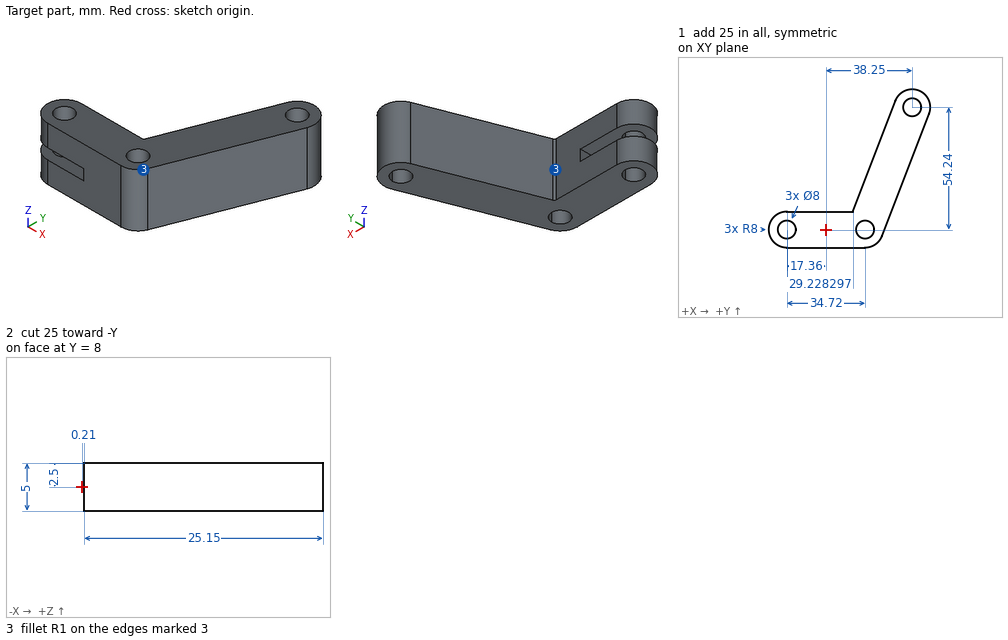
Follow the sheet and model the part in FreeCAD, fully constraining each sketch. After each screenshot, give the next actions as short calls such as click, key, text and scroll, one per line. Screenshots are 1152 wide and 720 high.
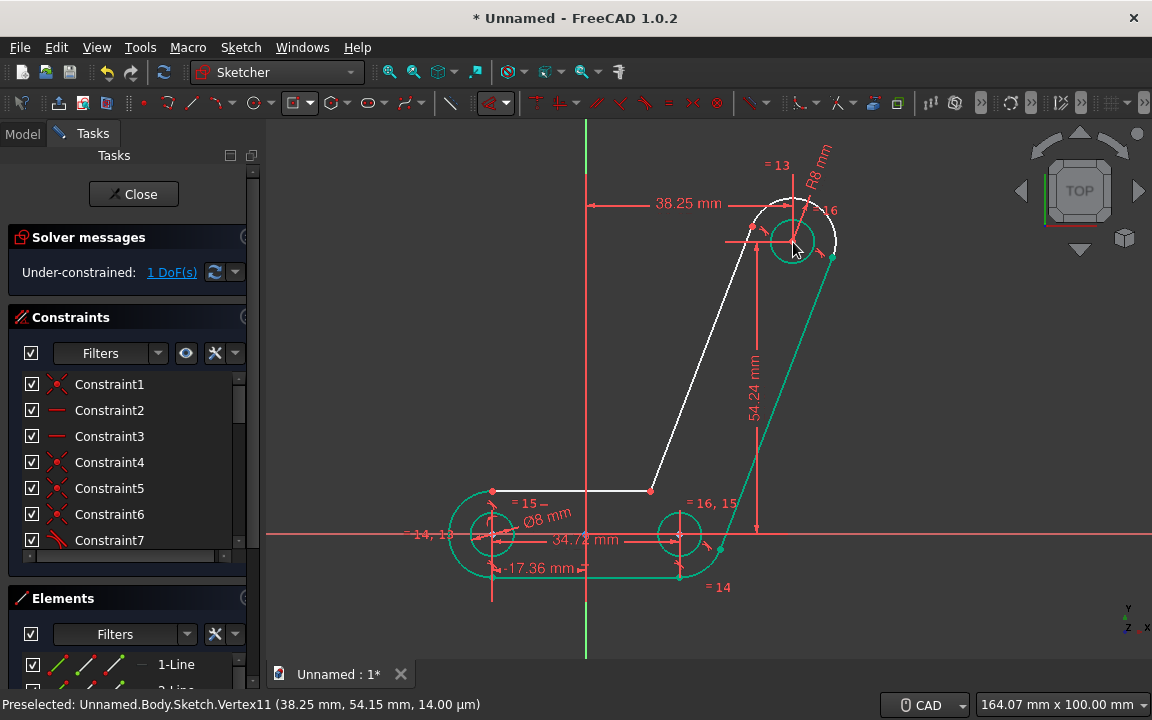
click(603, 491)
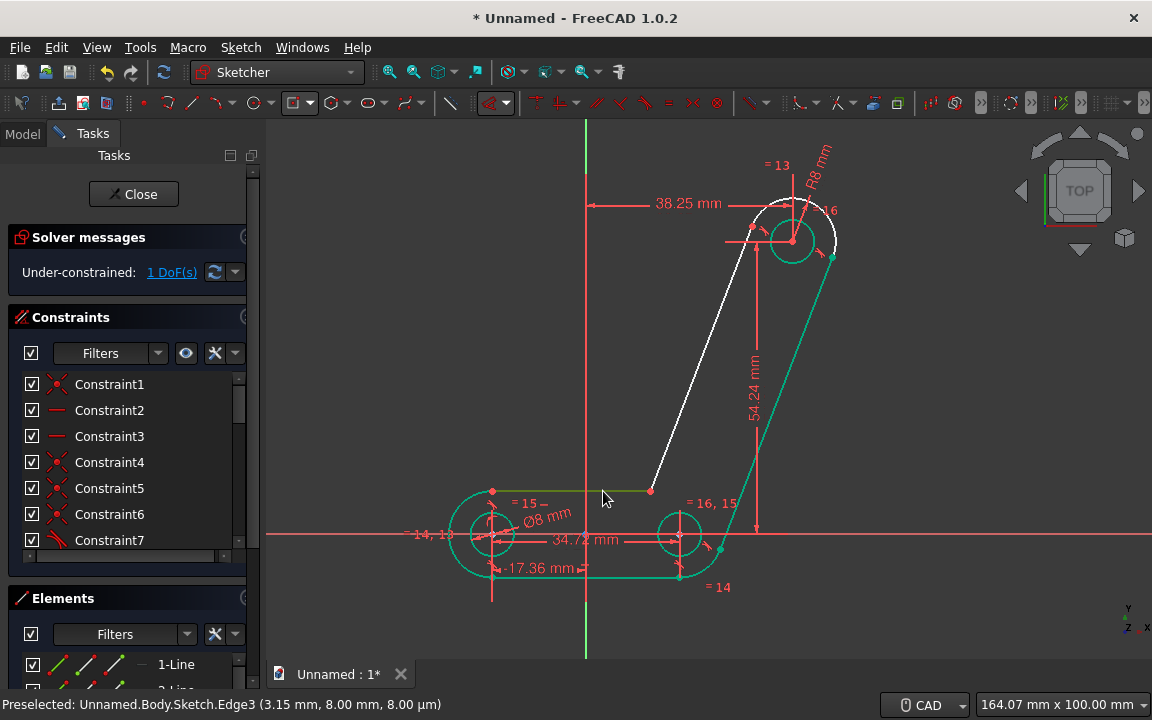
key(l)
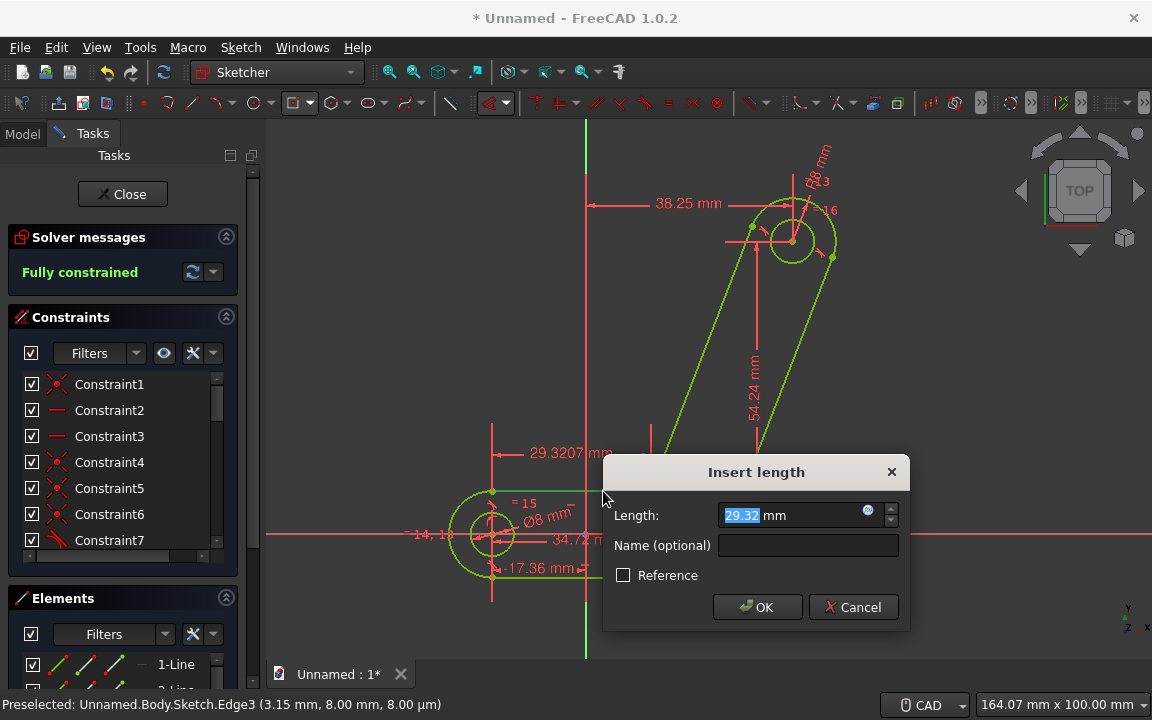
text(29.228297)
key(Return)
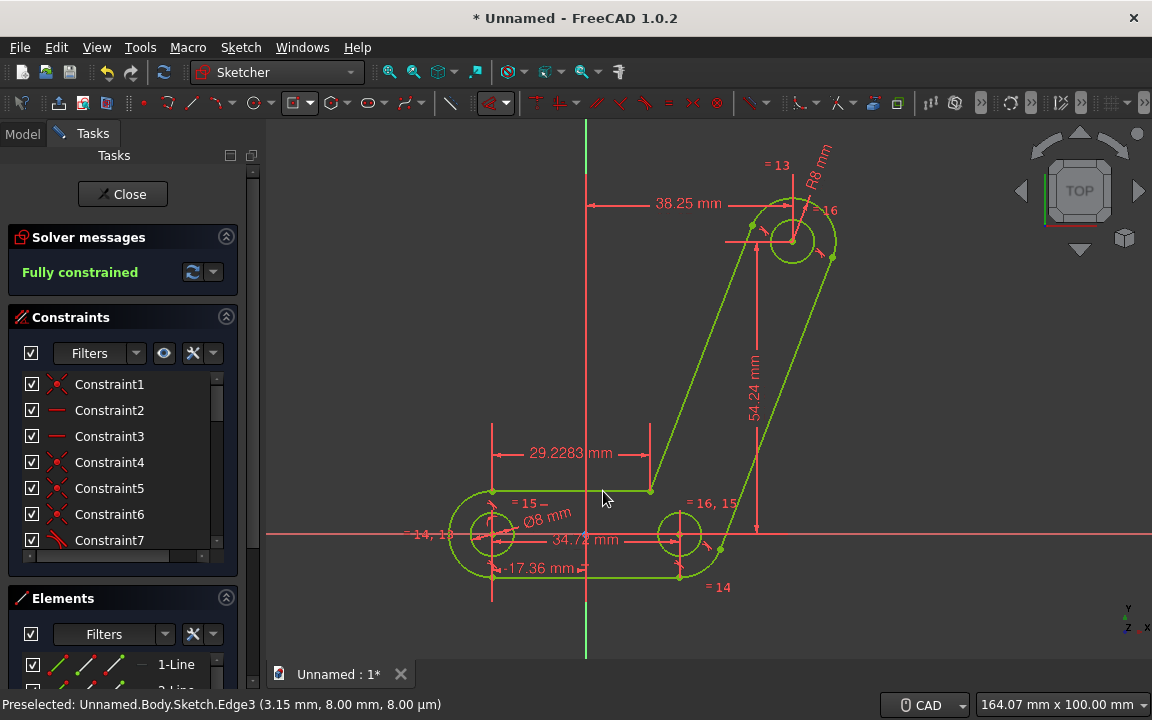
click(123, 194)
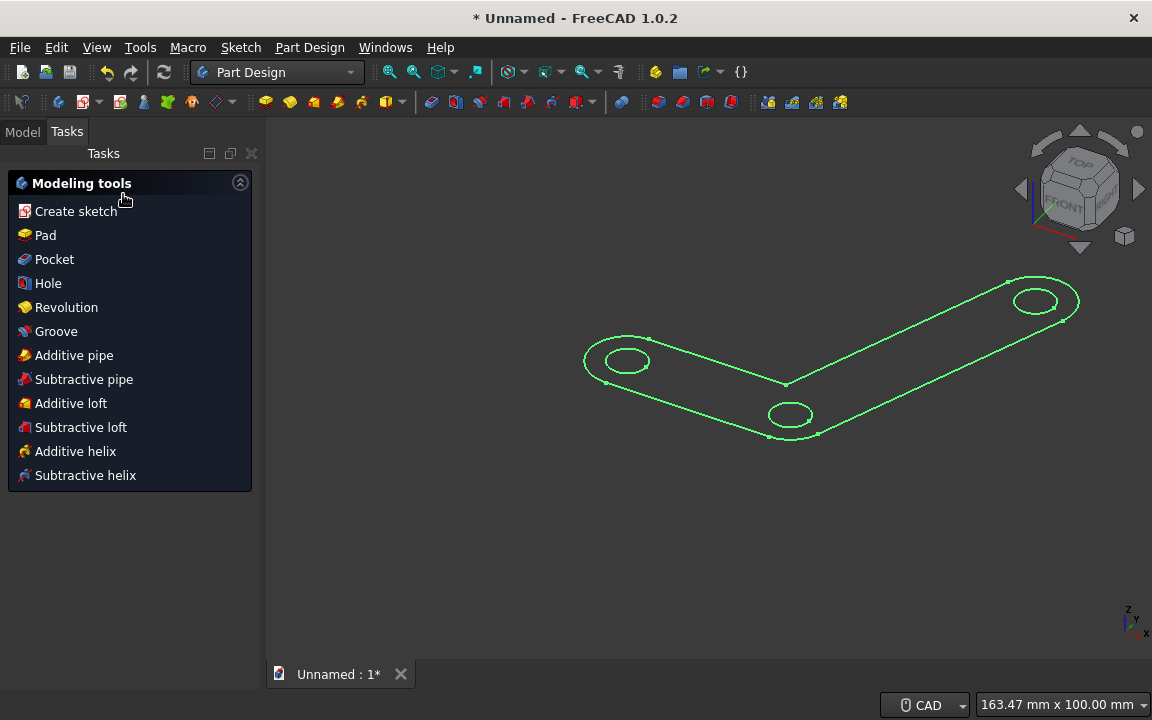
click(266, 102)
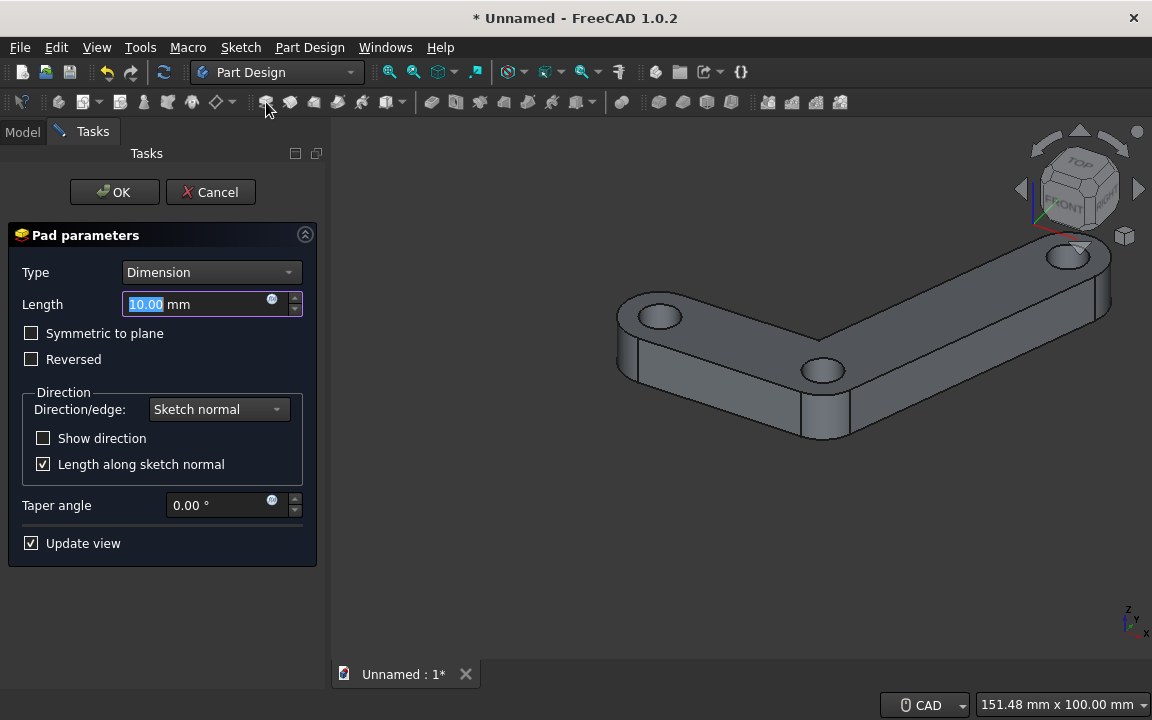
text(25)
key(Tab)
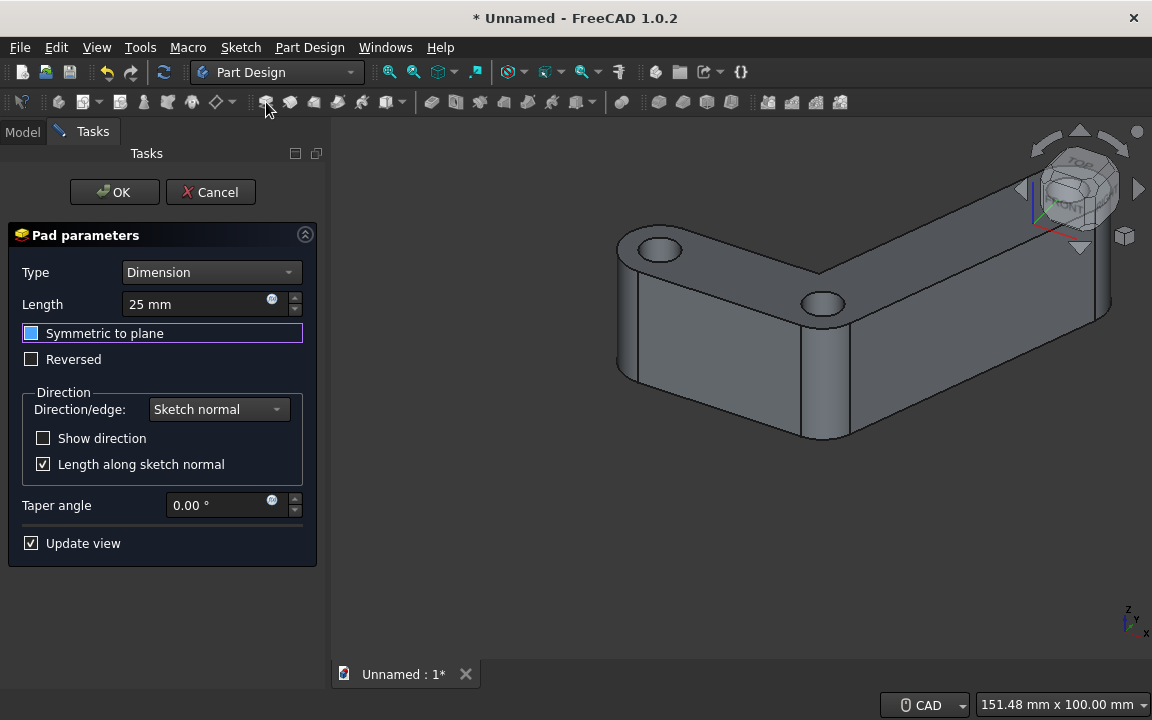
click(30, 333)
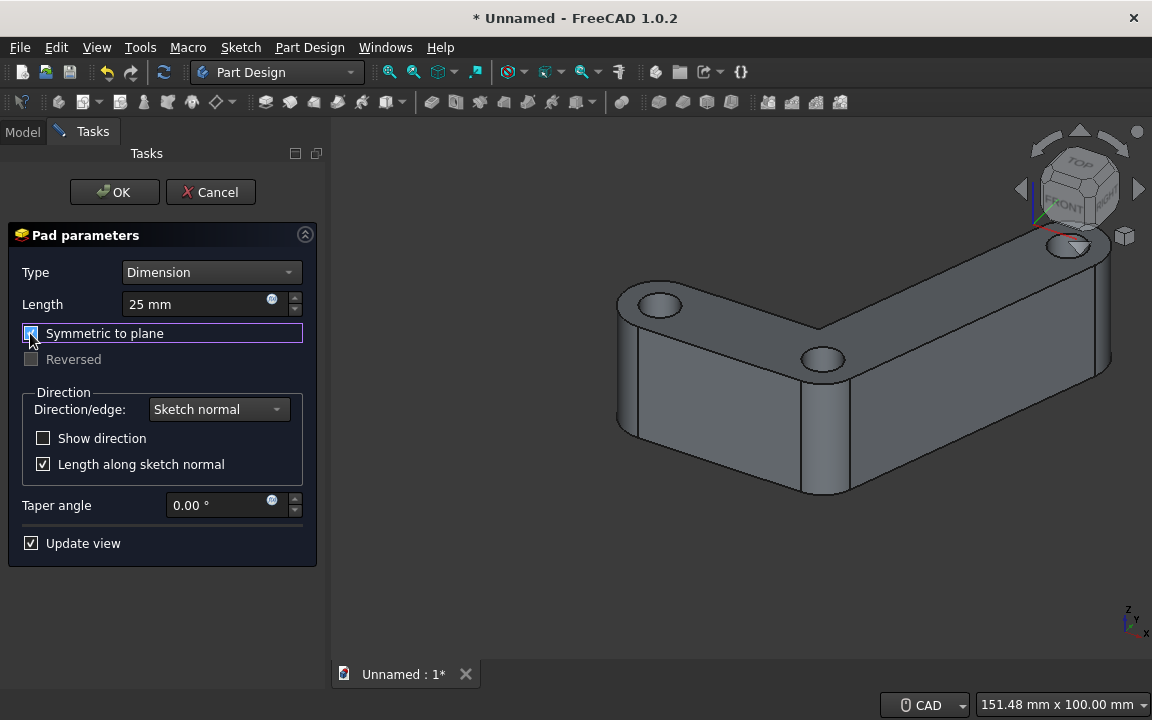
click(115, 192)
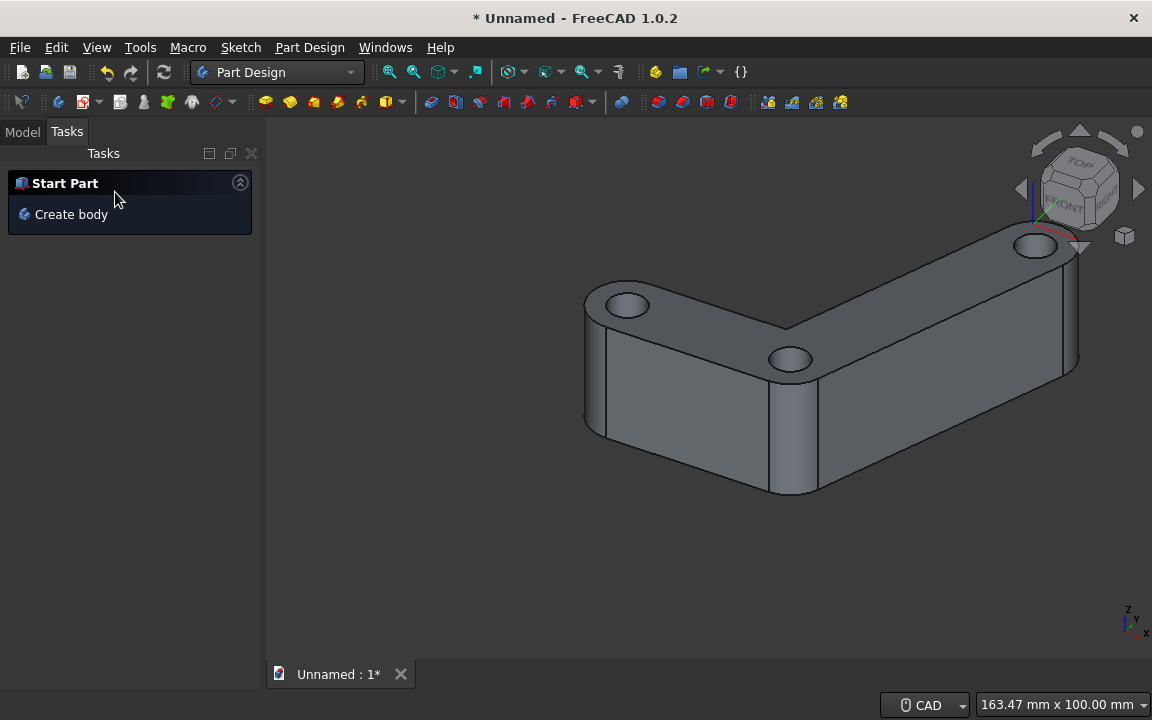
key(4)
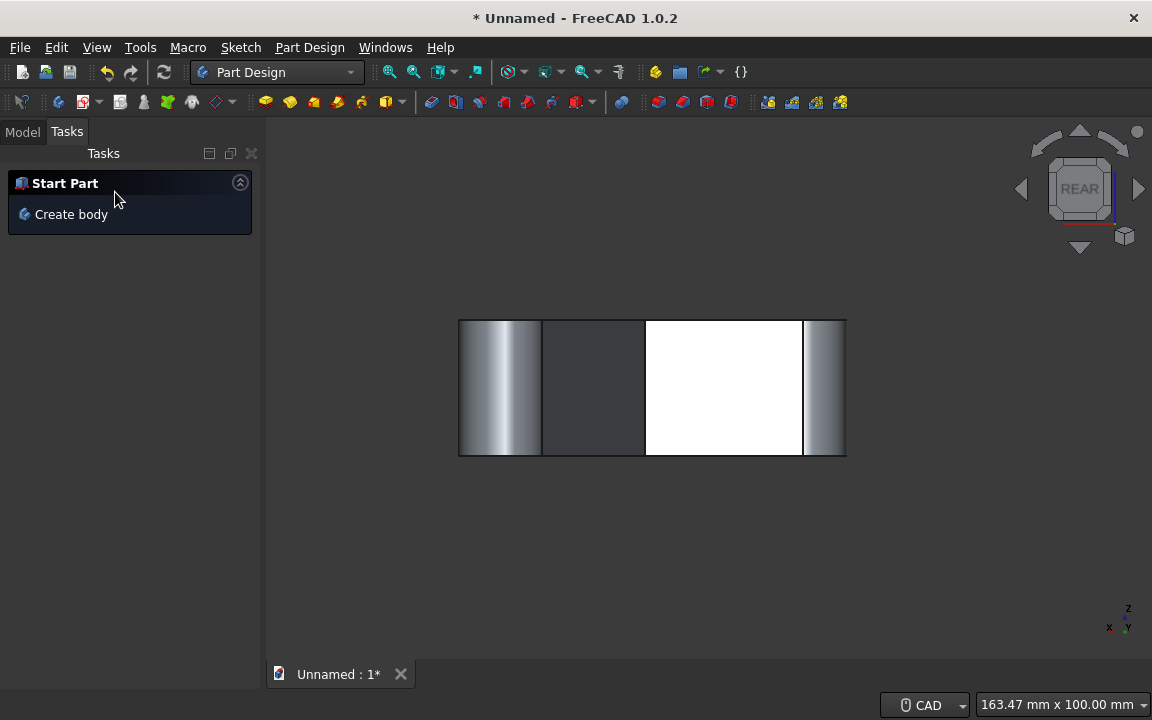
click(390, 72)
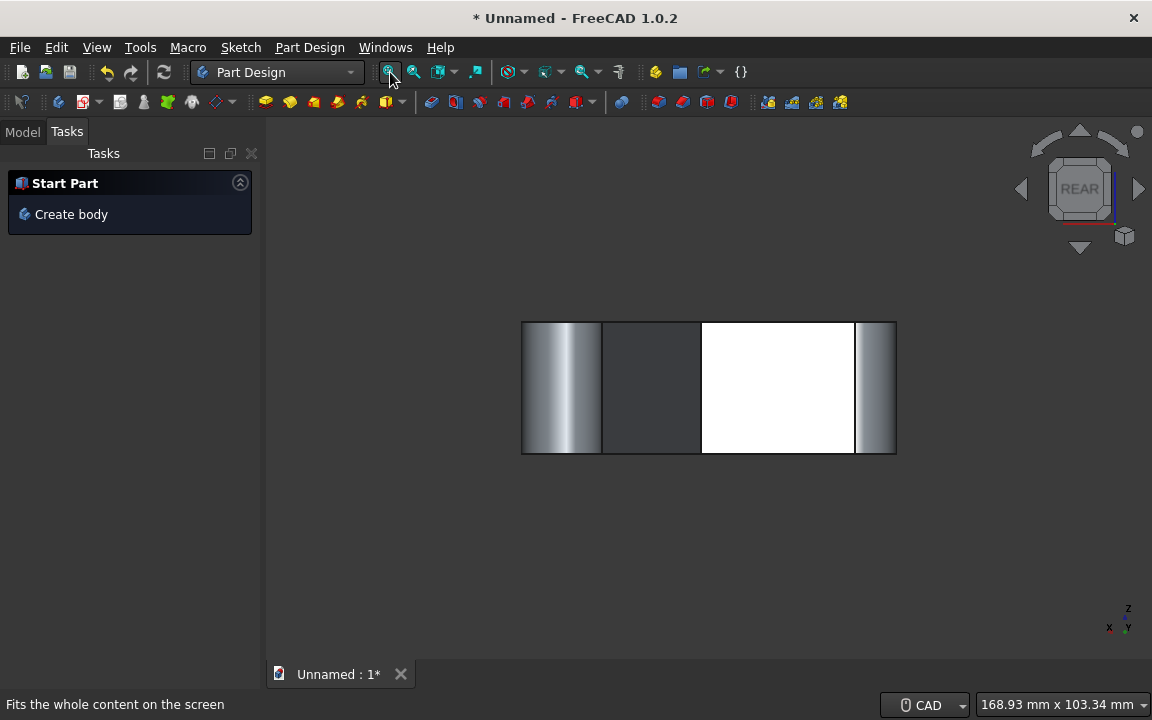
click(778, 387)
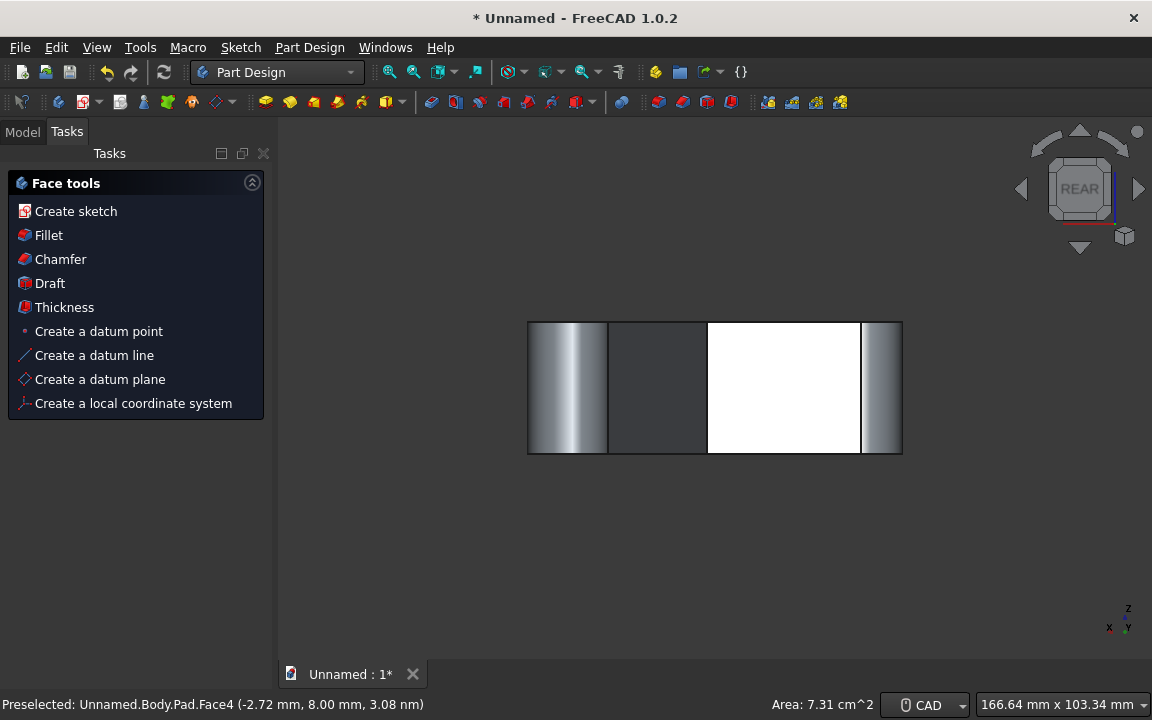
click(84, 102)